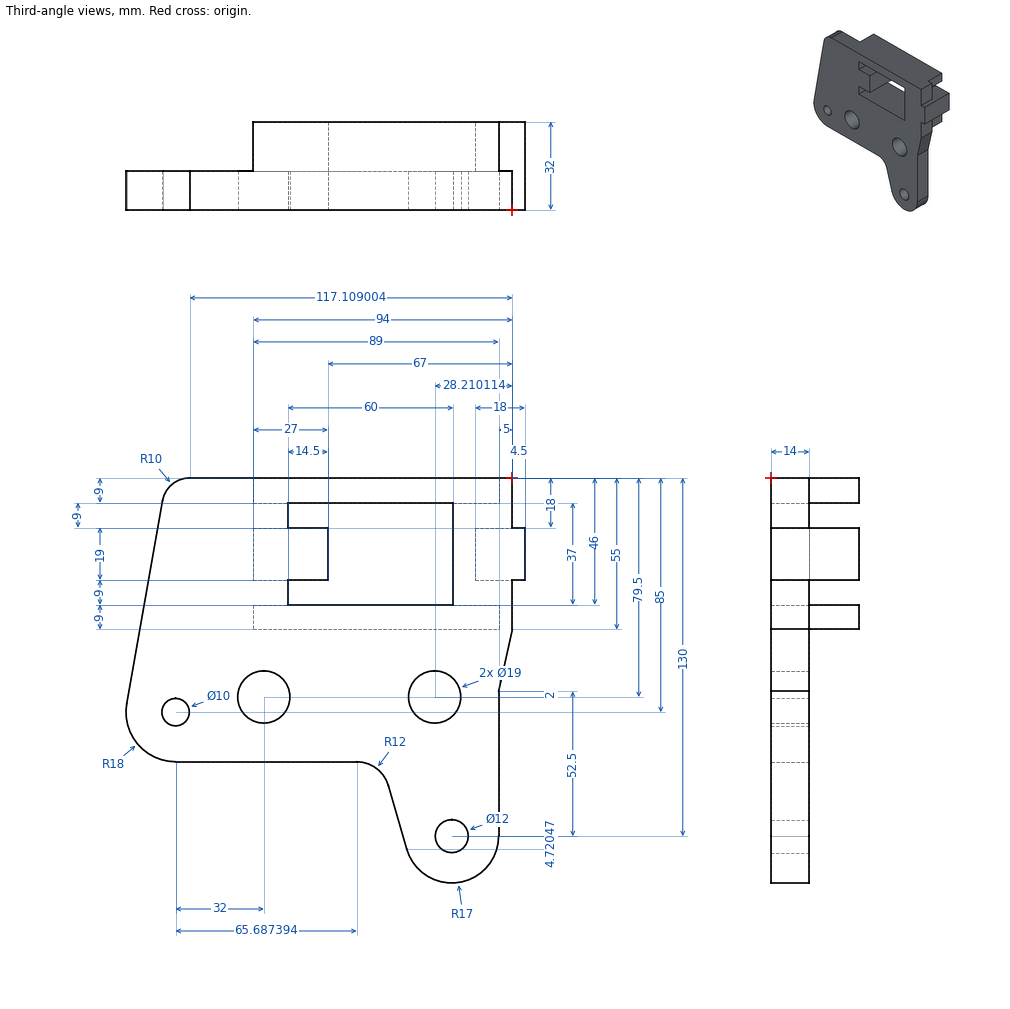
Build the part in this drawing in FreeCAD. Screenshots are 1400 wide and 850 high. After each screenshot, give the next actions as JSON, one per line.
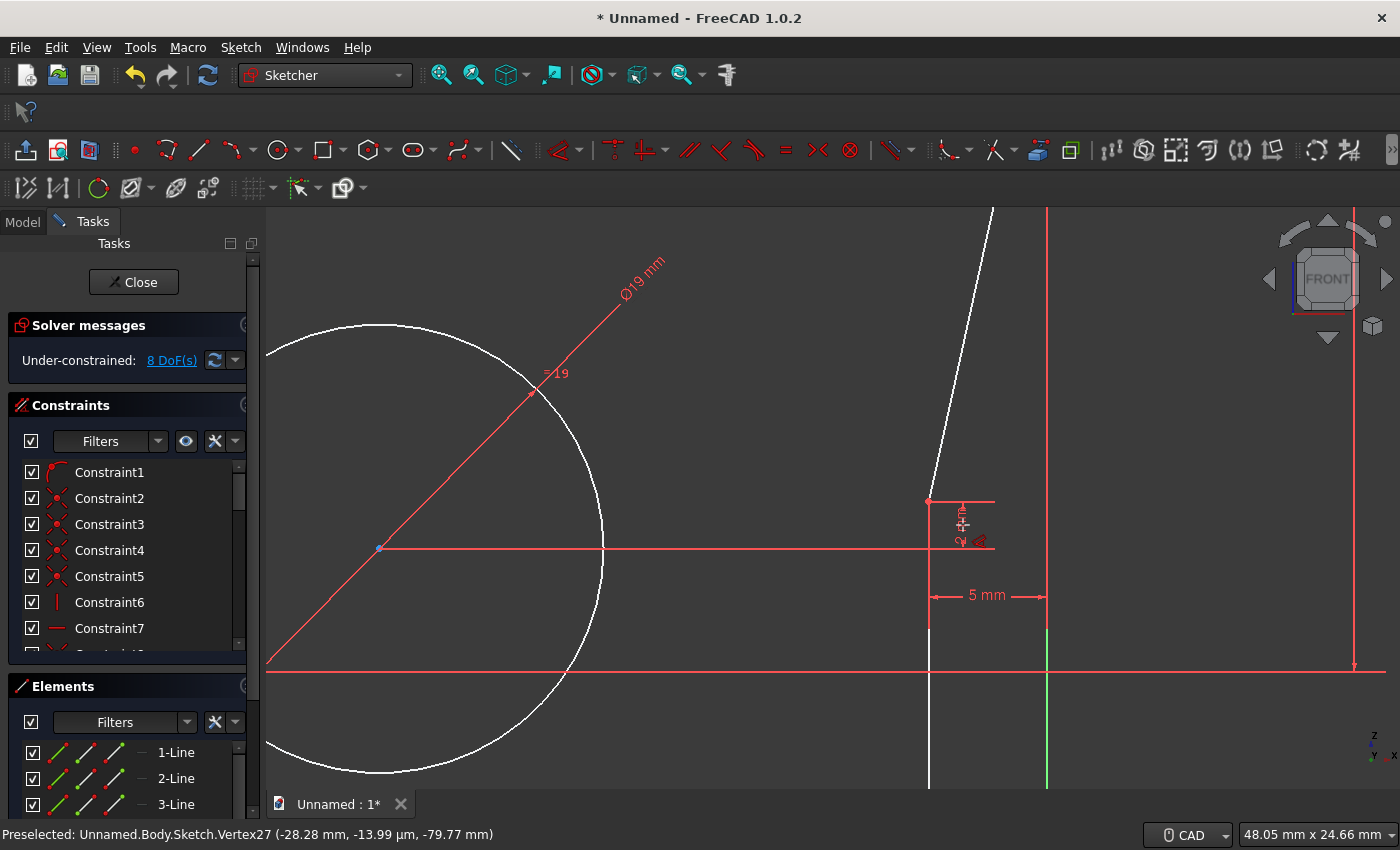
{"action": "scroll", "coordinate": [935, 510], "scroll_direction": "down", "scroll_amount": 11}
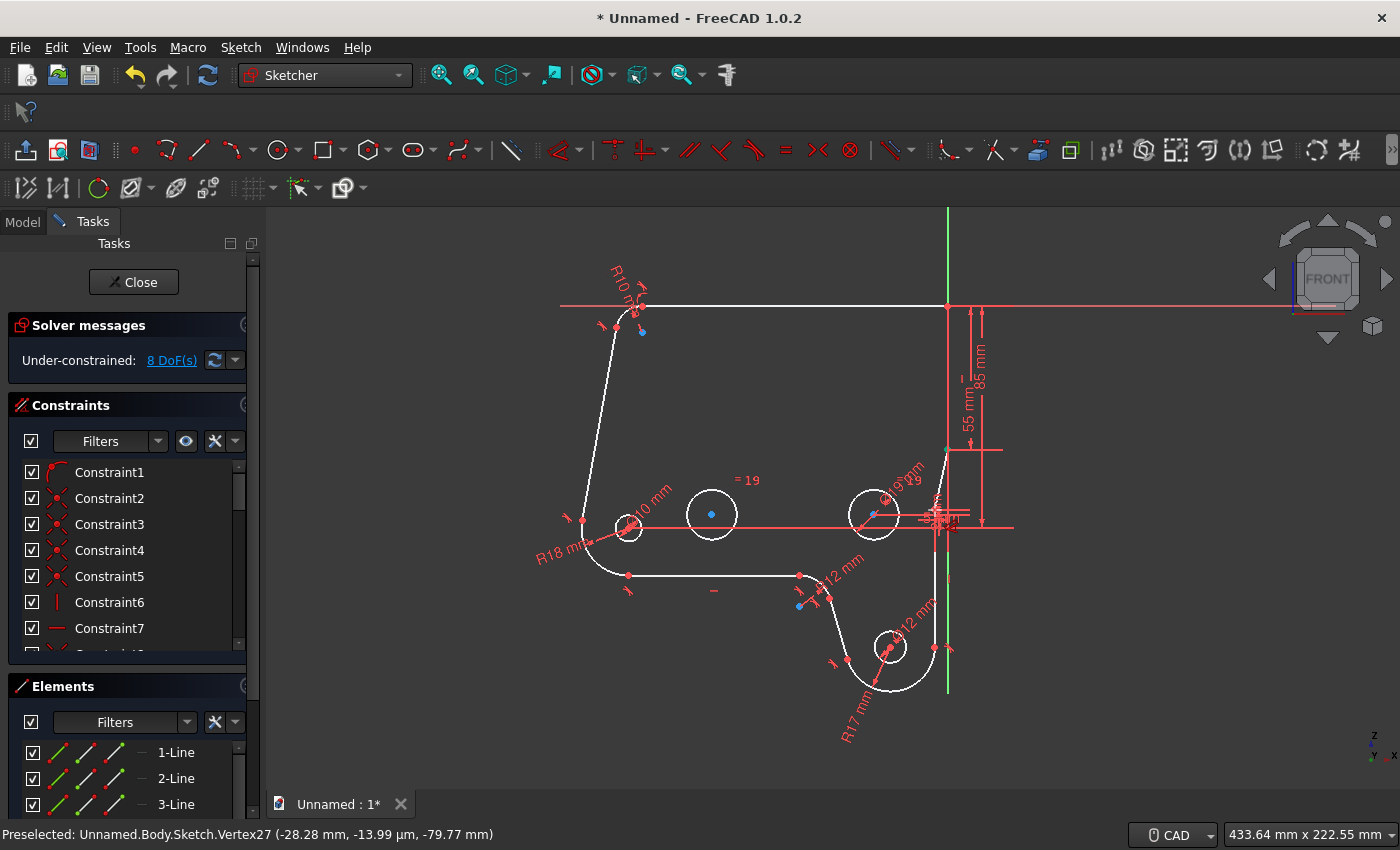
{"action": "left_click", "coordinate": [890, 647]}
{"action": "left_click", "coordinate": [982, 477]}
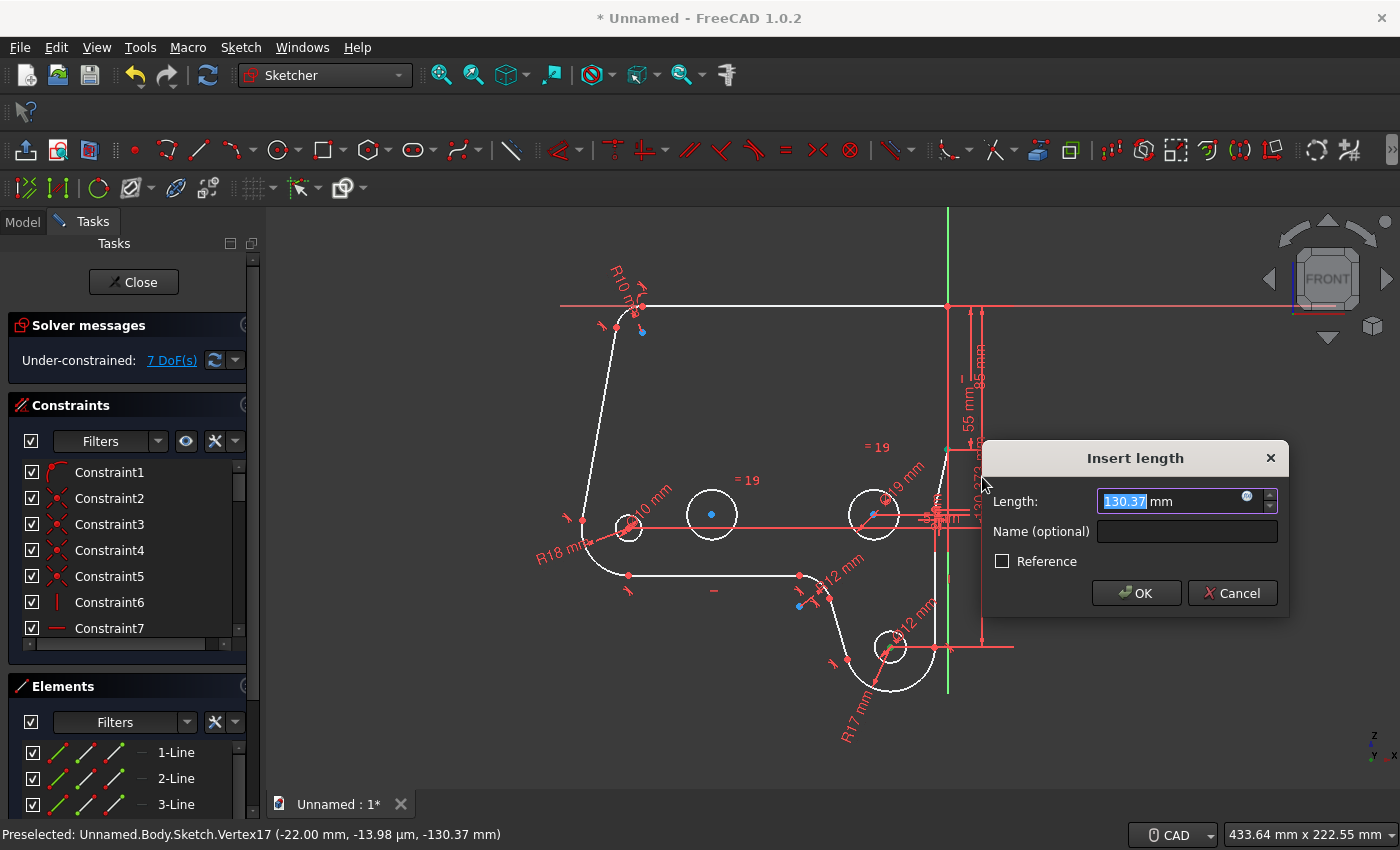
{"action": "type", "text": "130"}
{"action": "key", "text": "Return"}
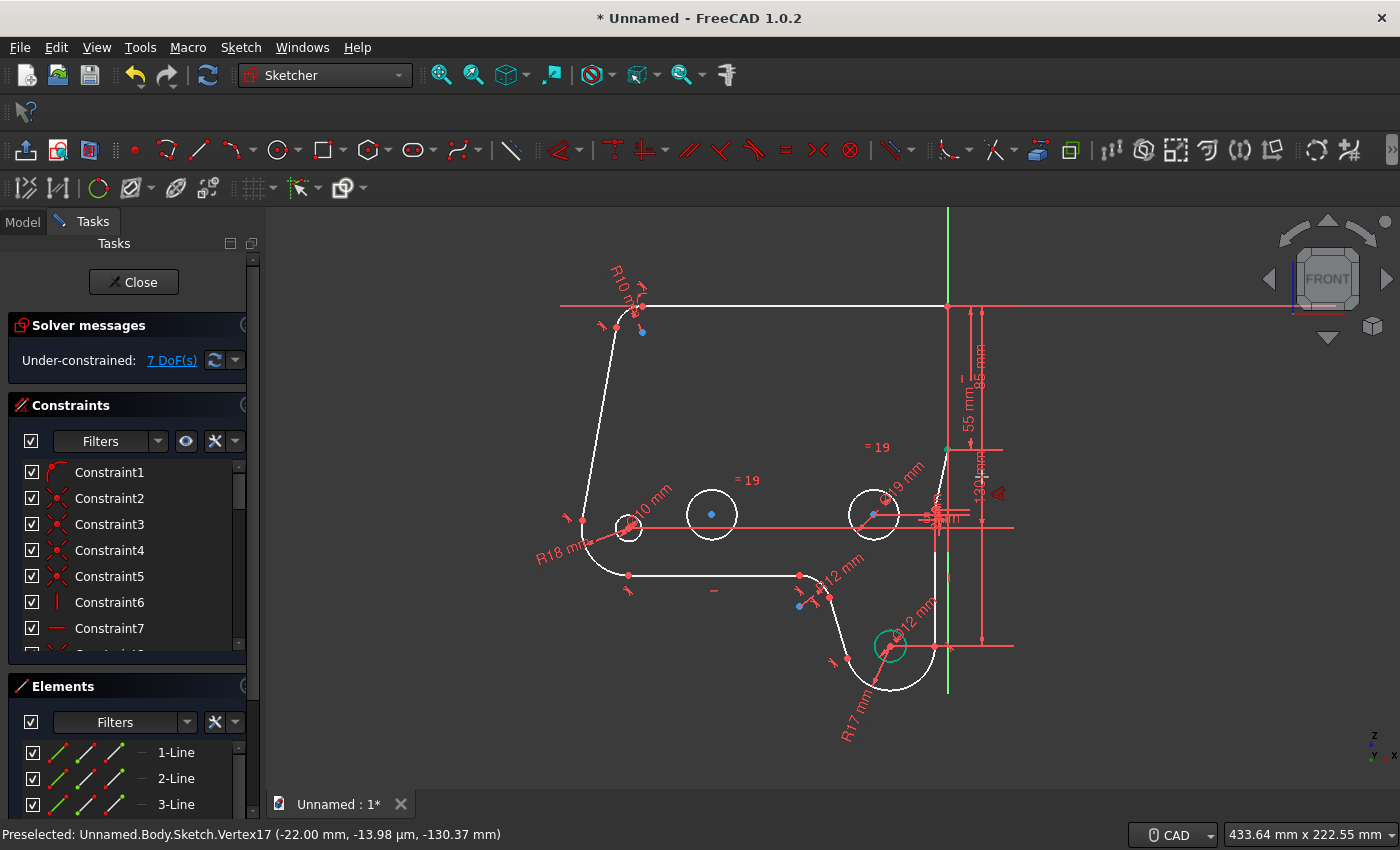
{"action": "left_click", "coordinate": [629, 576]}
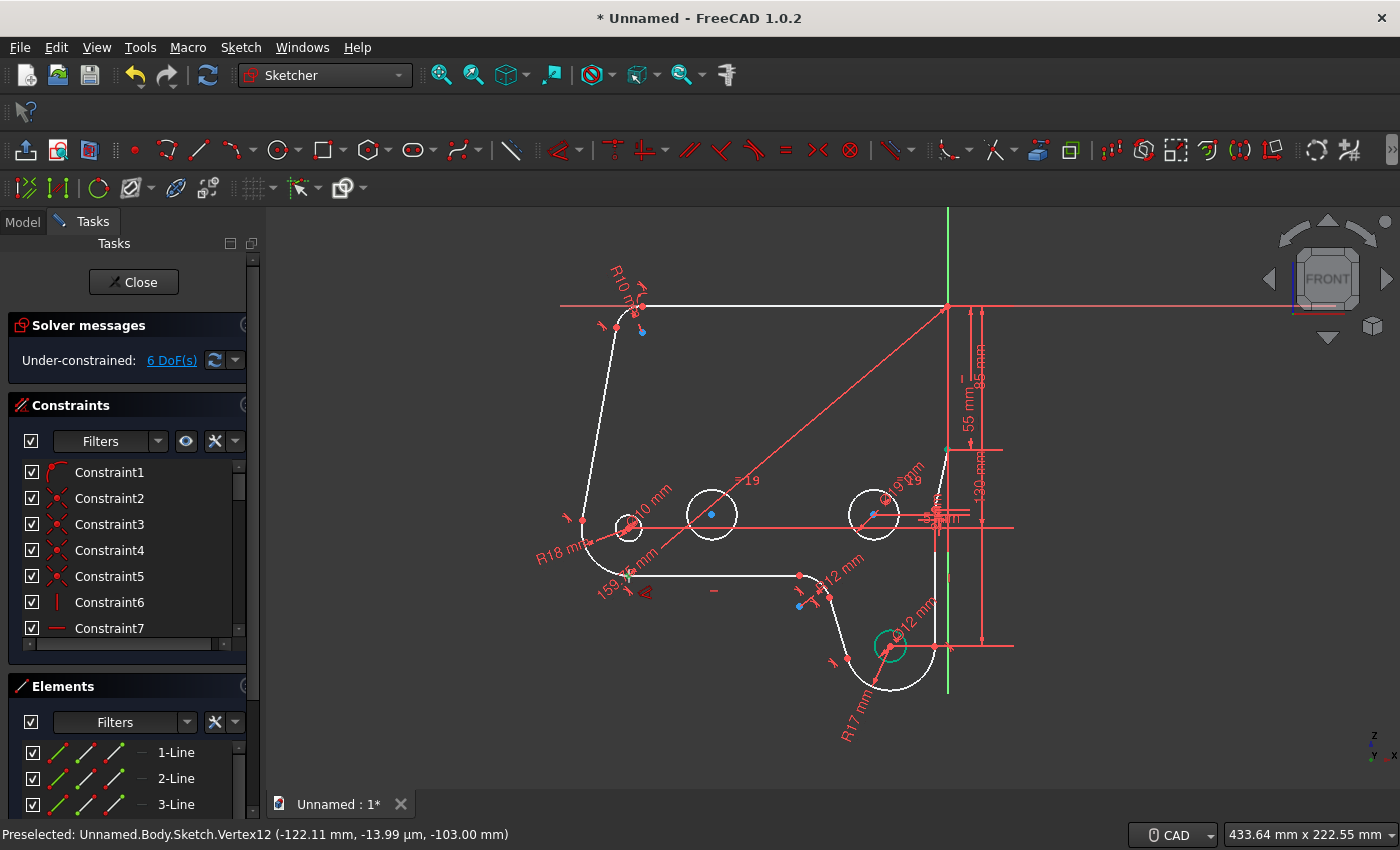
{"action": "left_click", "coordinate": [712, 515]}
{"action": "left_click", "coordinate": [670, 610]}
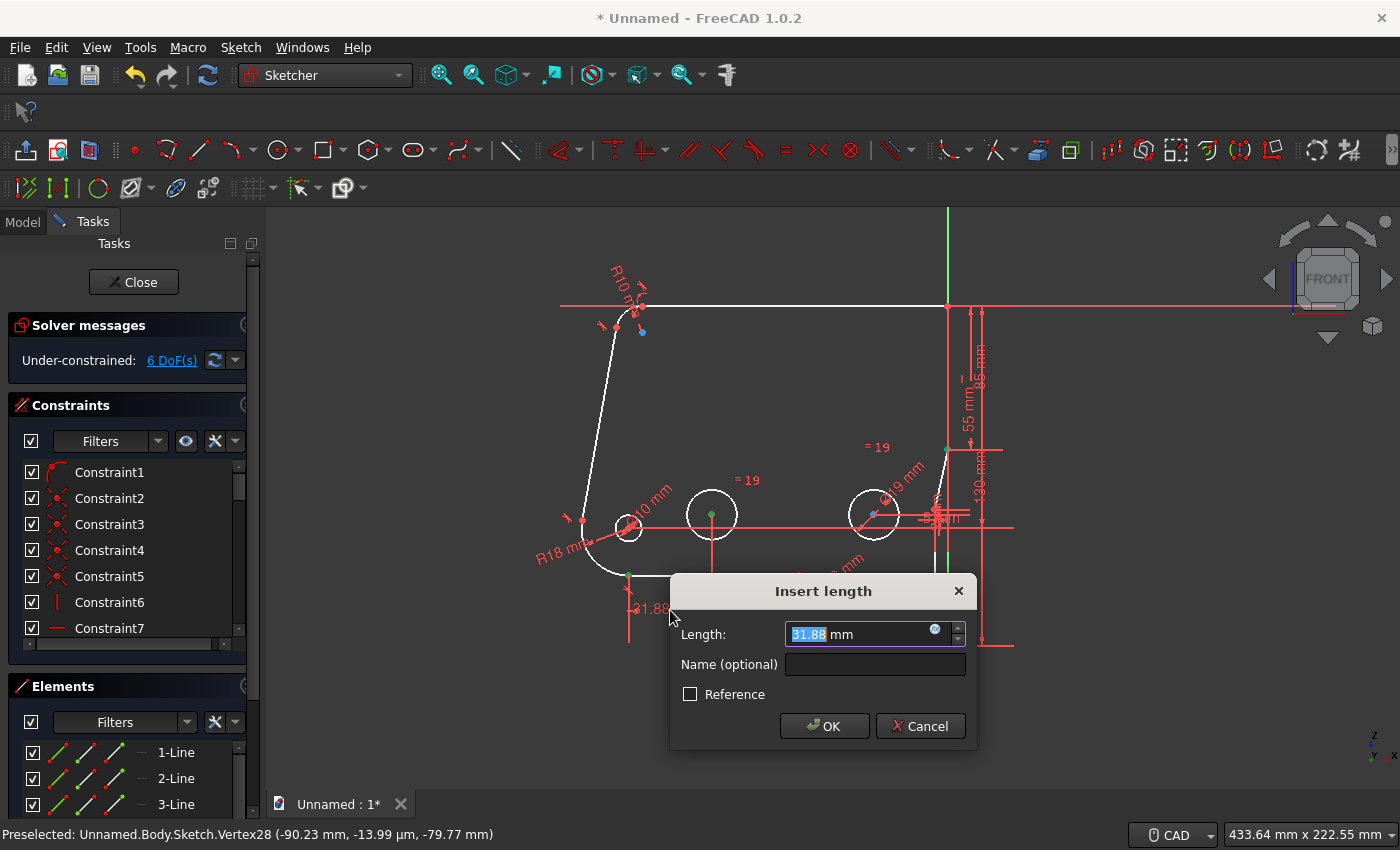
{"action": "type", "text": "32"}
{"action": "key", "text": "Return"}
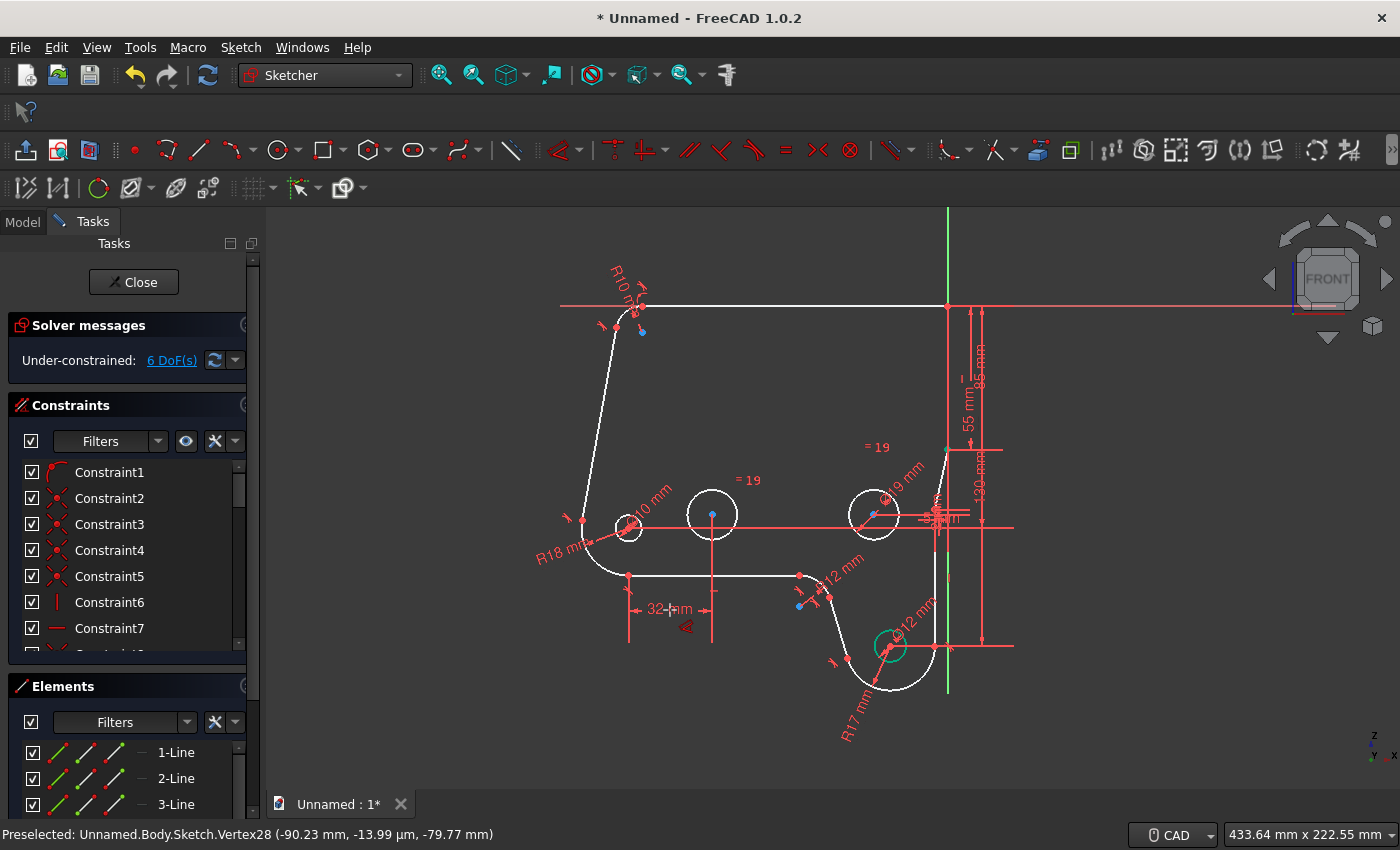
{"action": "left_click", "coordinate": [935, 551]}
{"action": "left_click", "coordinate": [969, 578]}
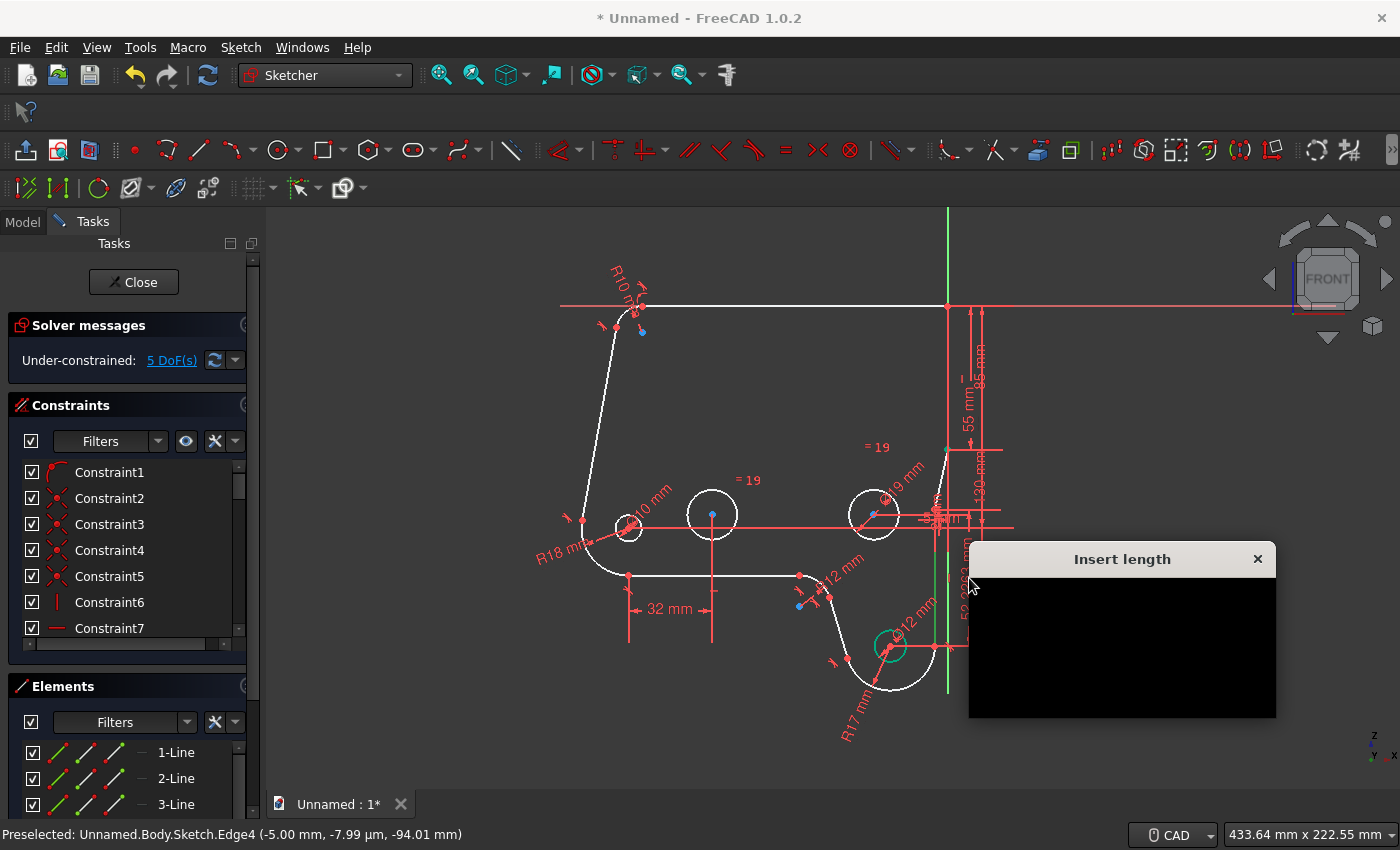
{"action": "type", "text": "52.5"}
{"action": "key", "text": "Return"}